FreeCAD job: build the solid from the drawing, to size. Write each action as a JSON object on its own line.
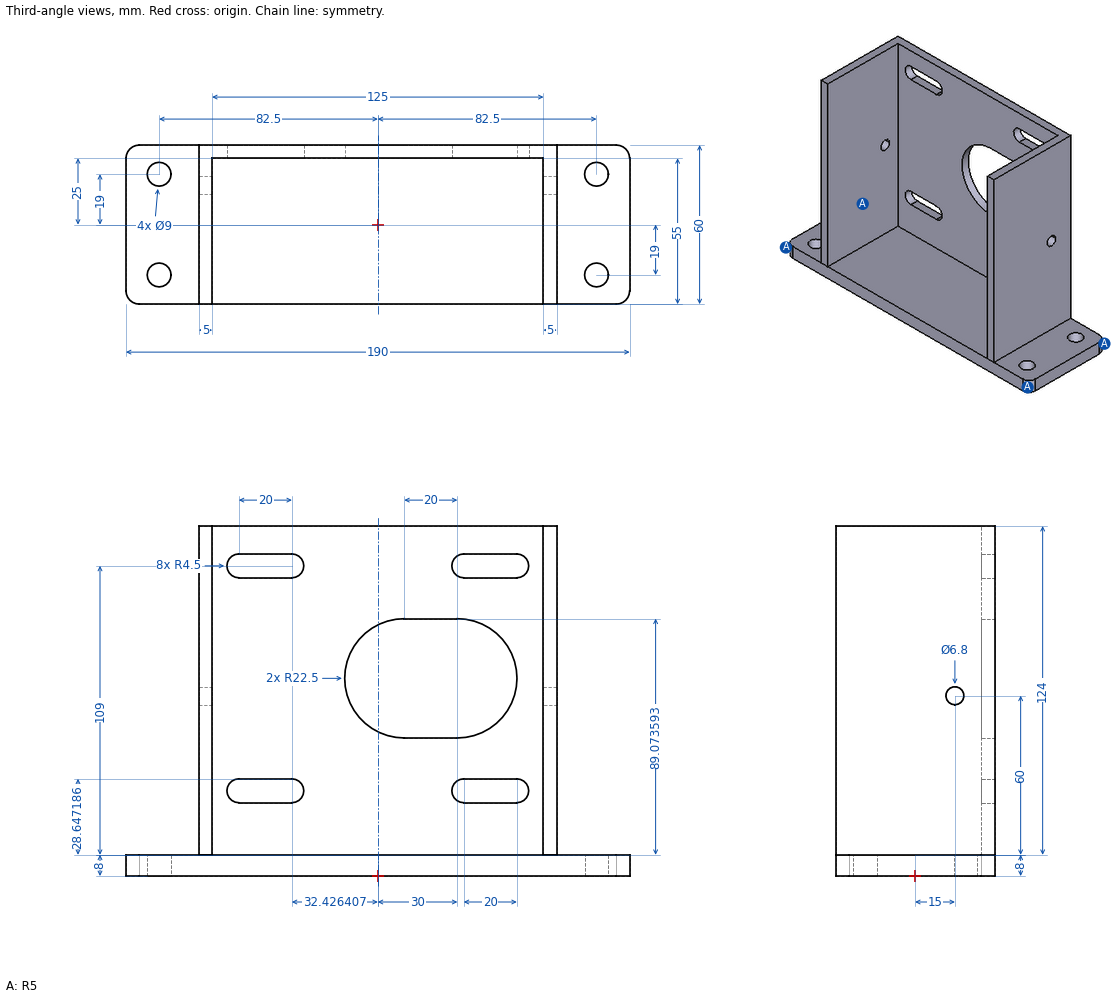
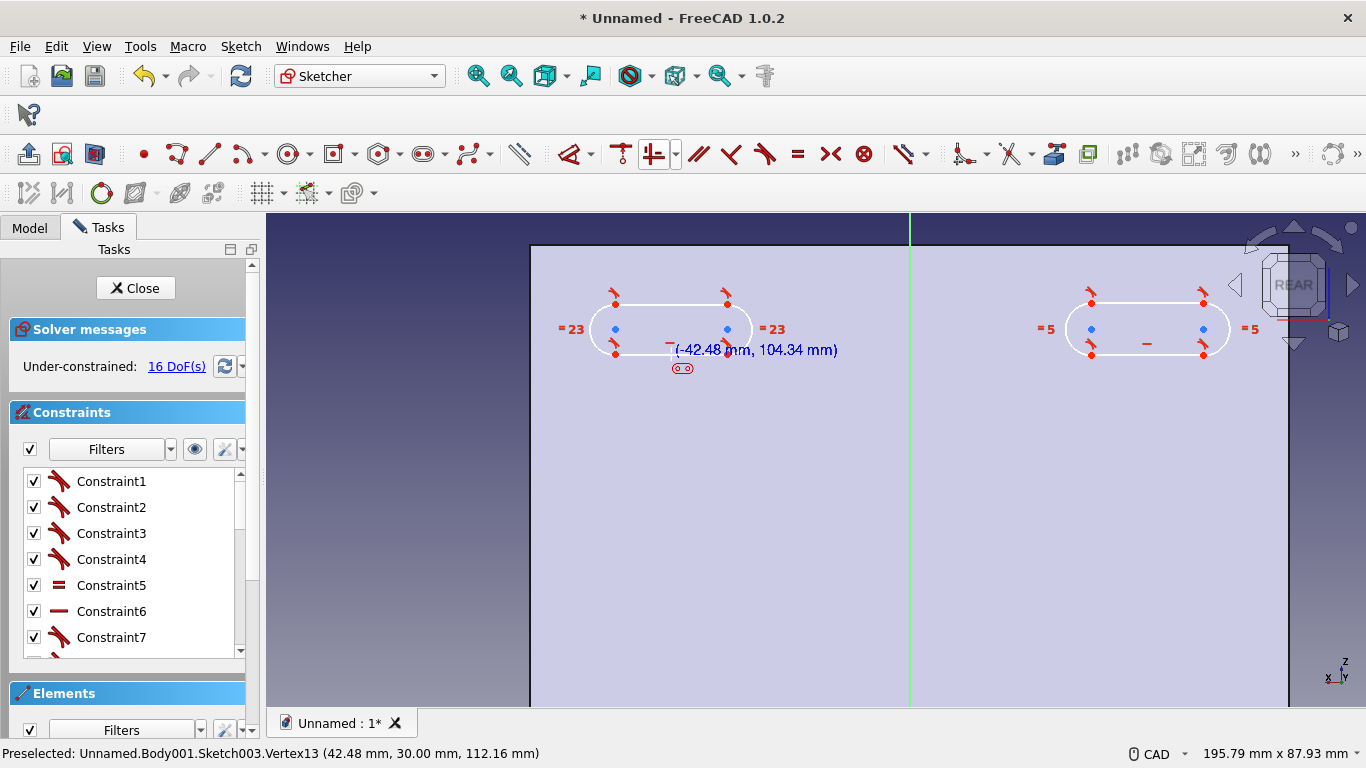
{"action": "left_click", "coordinate": [741, 567]}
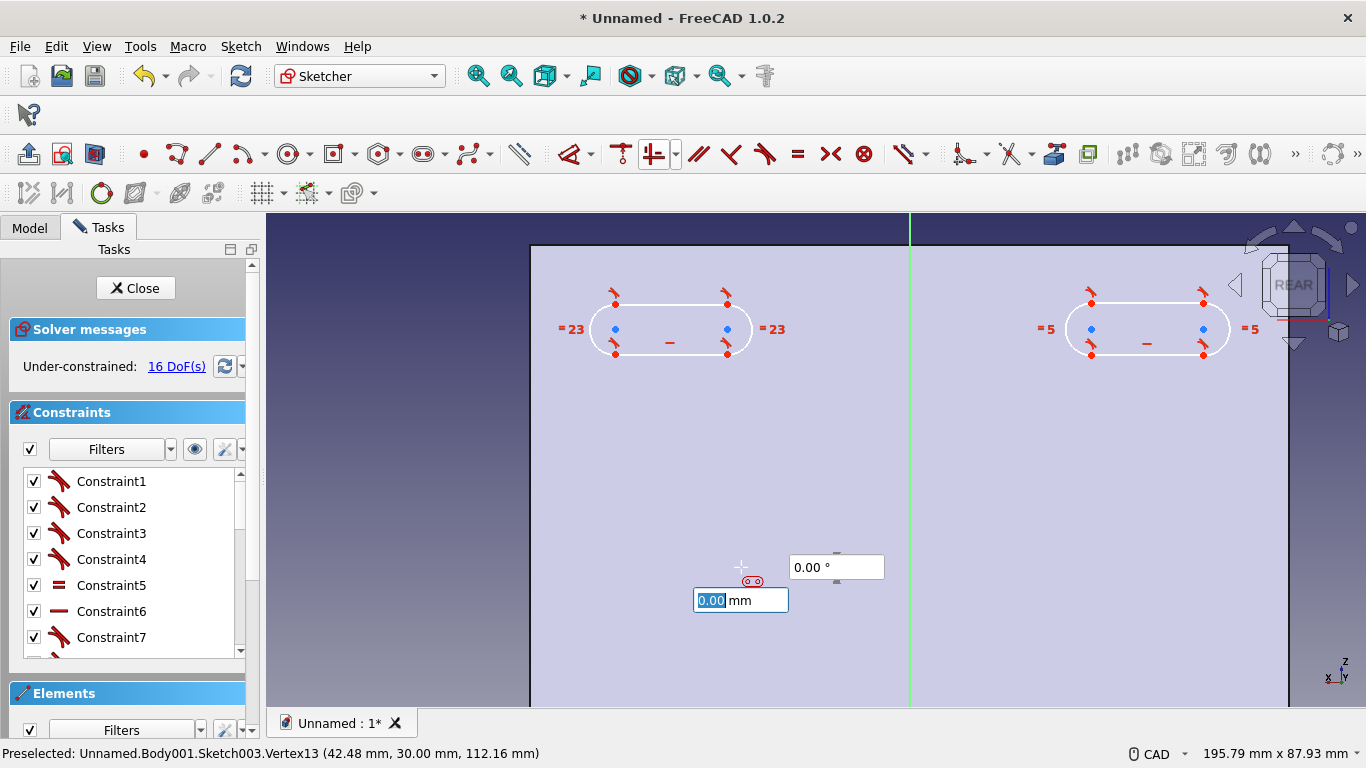
{"action": "left_click", "coordinate": [853, 567]}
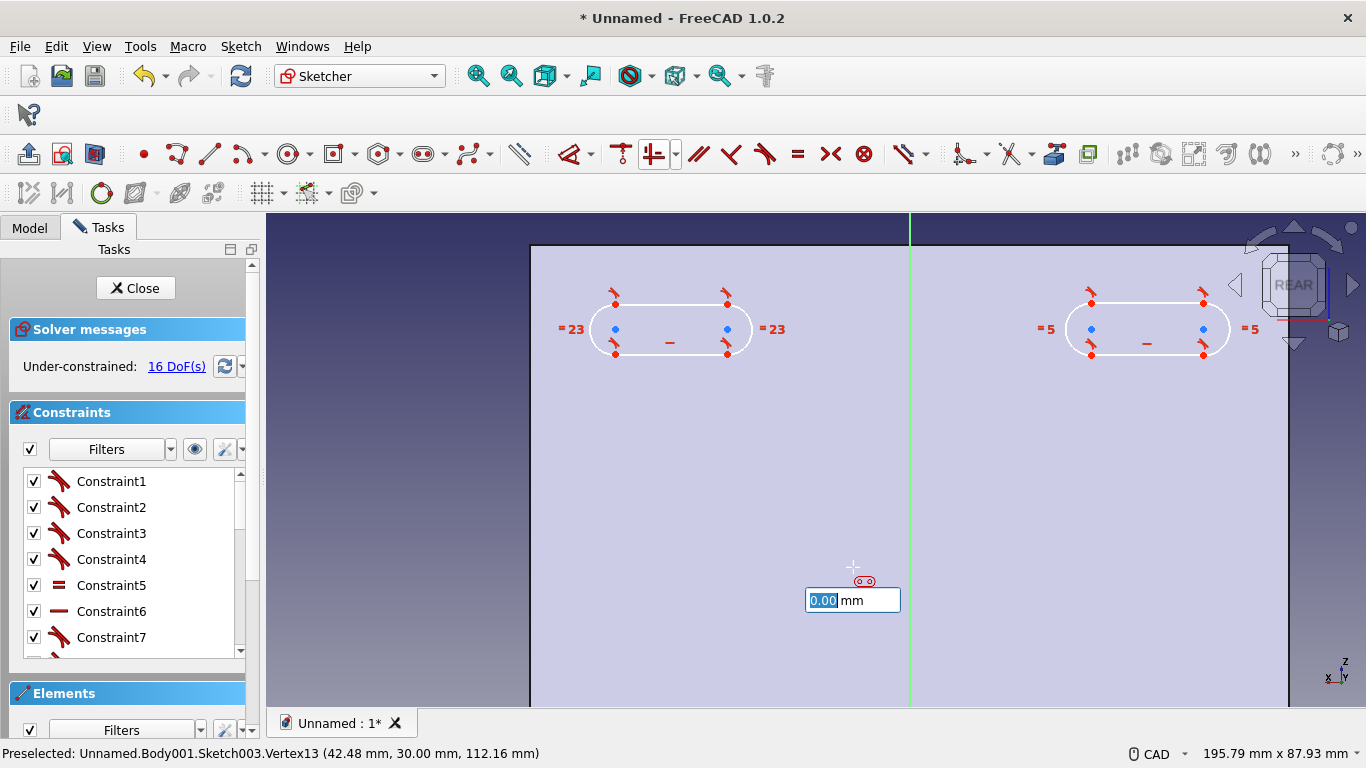
{"action": "scroll", "coordinate": [615, 327], "scroll_direction": "down", "scroll_amount": 4}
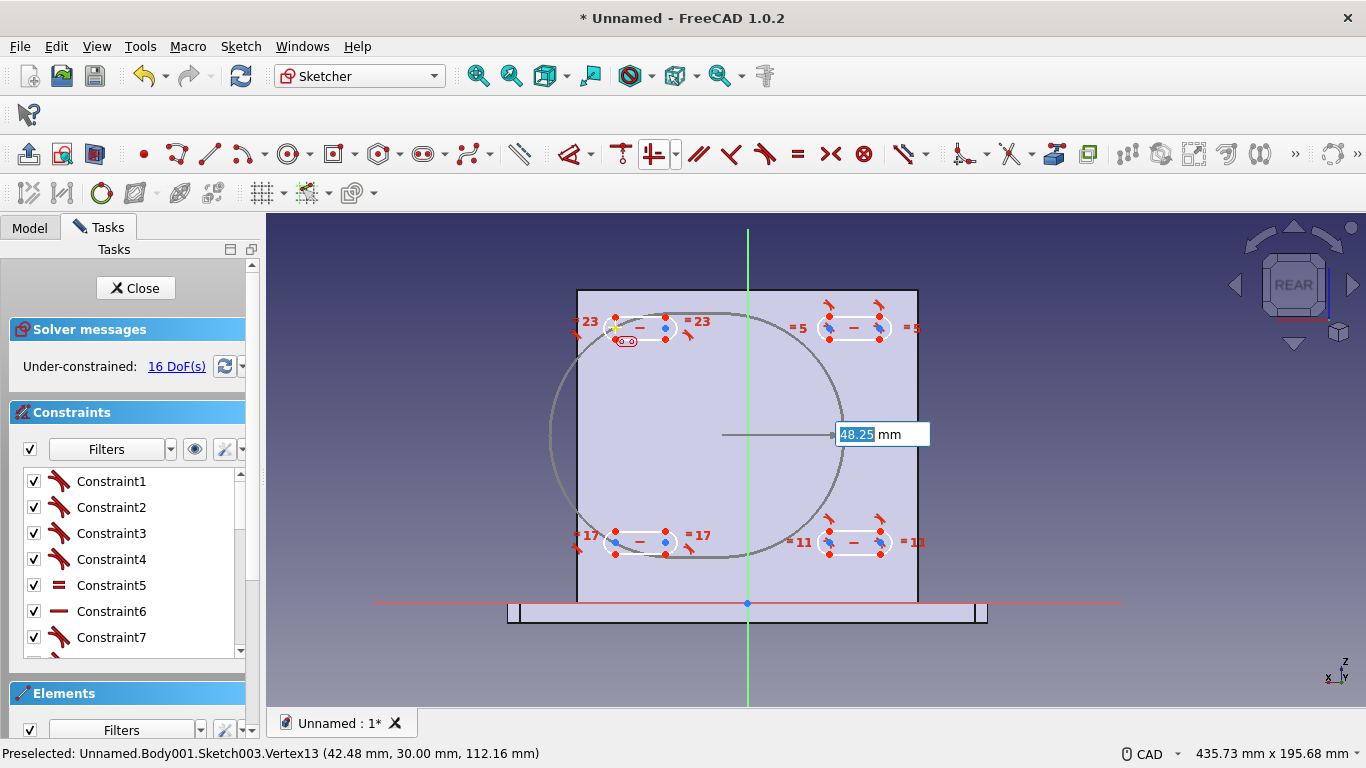
{"action": "left_click", "coordinate": [697, 492]}
{"action": "key", "text": "Escape"}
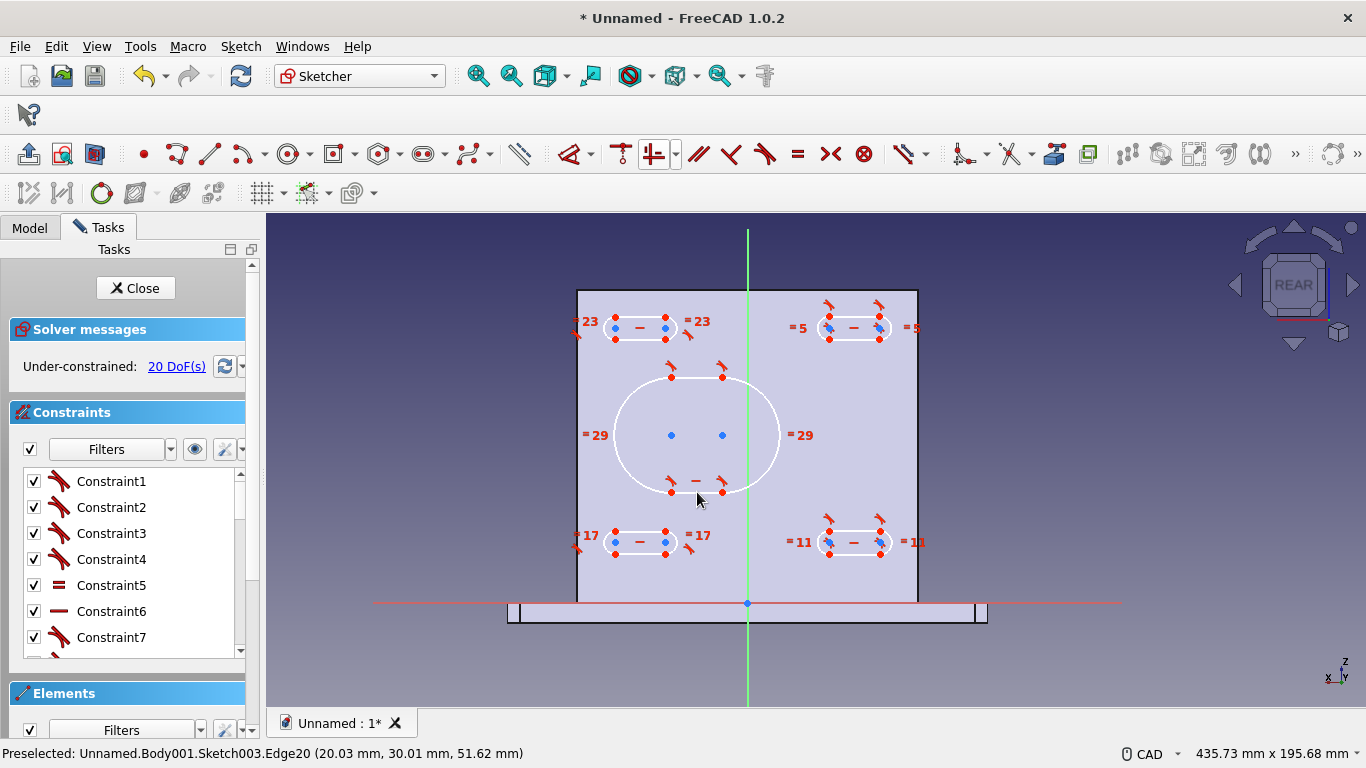
{"action": "scroll", "coordinate": [820, 321], "scroll_direction": "up", "scroll_amount": 2}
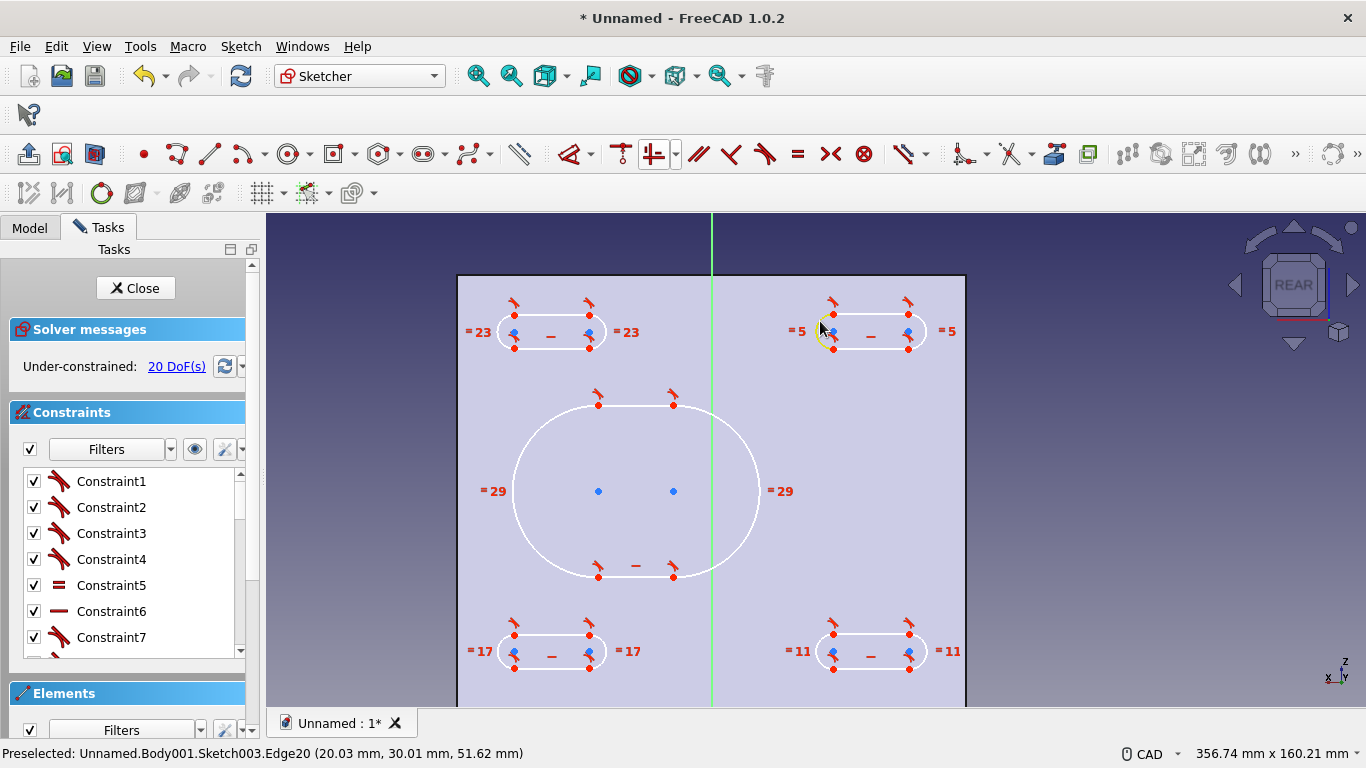
{"action": "left_click", "coordinate": [820, 321]}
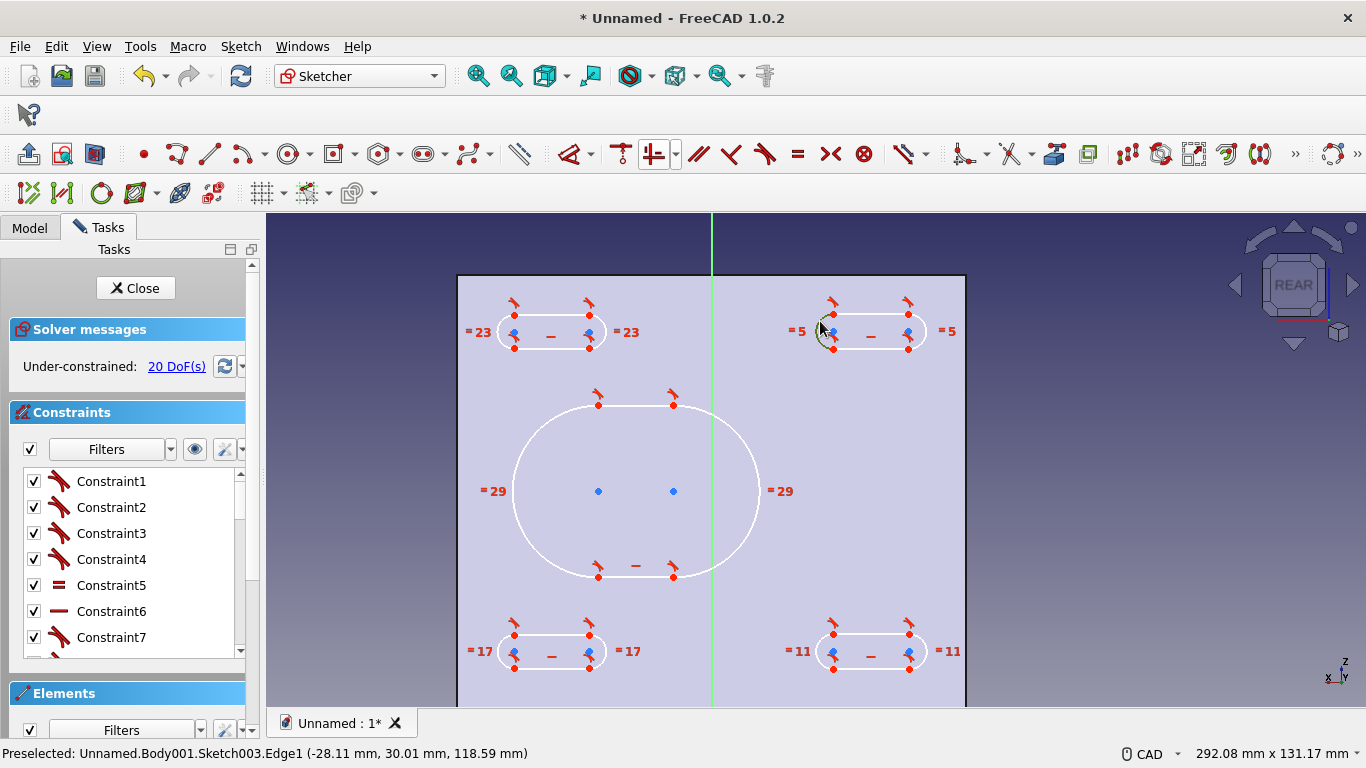
{"action": "left_click", "coordinate": [819, 642]}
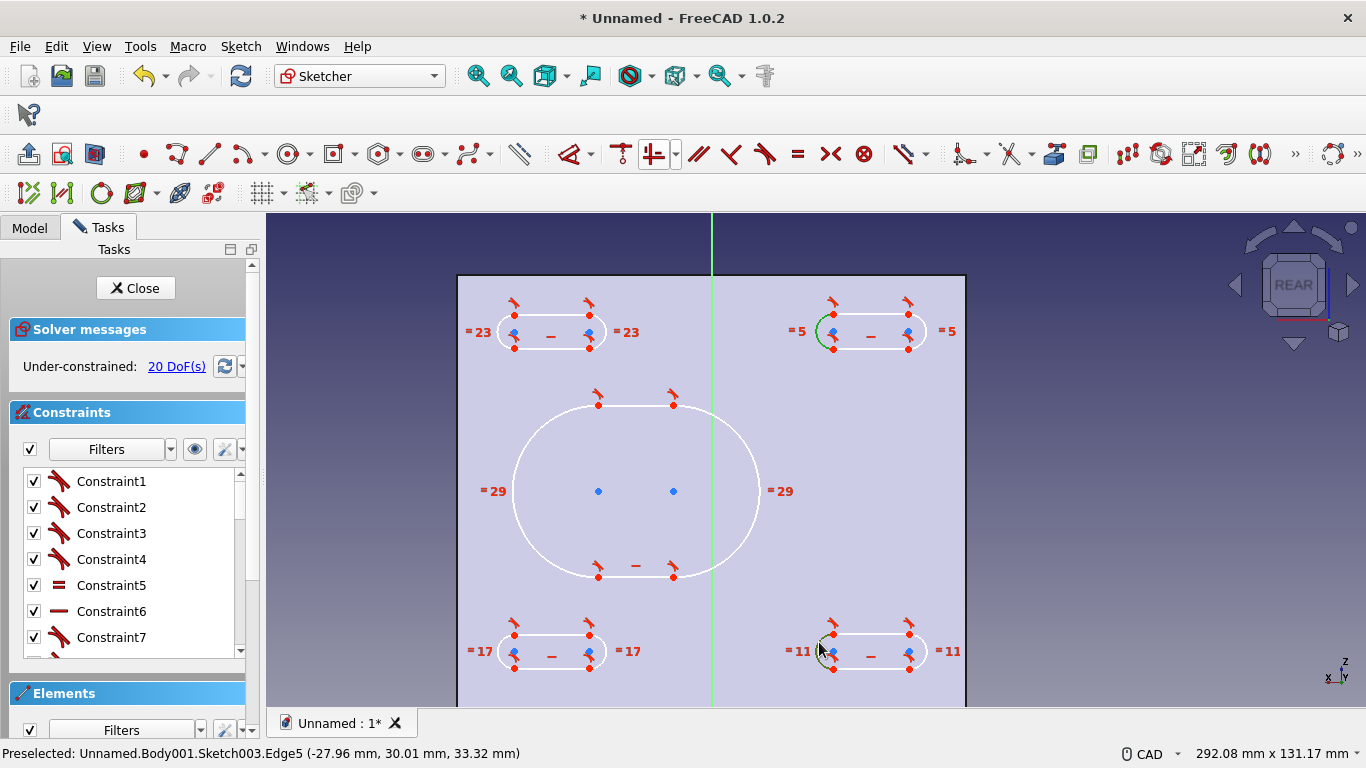
{"action": "left_click", "coordinate": [501, 642]}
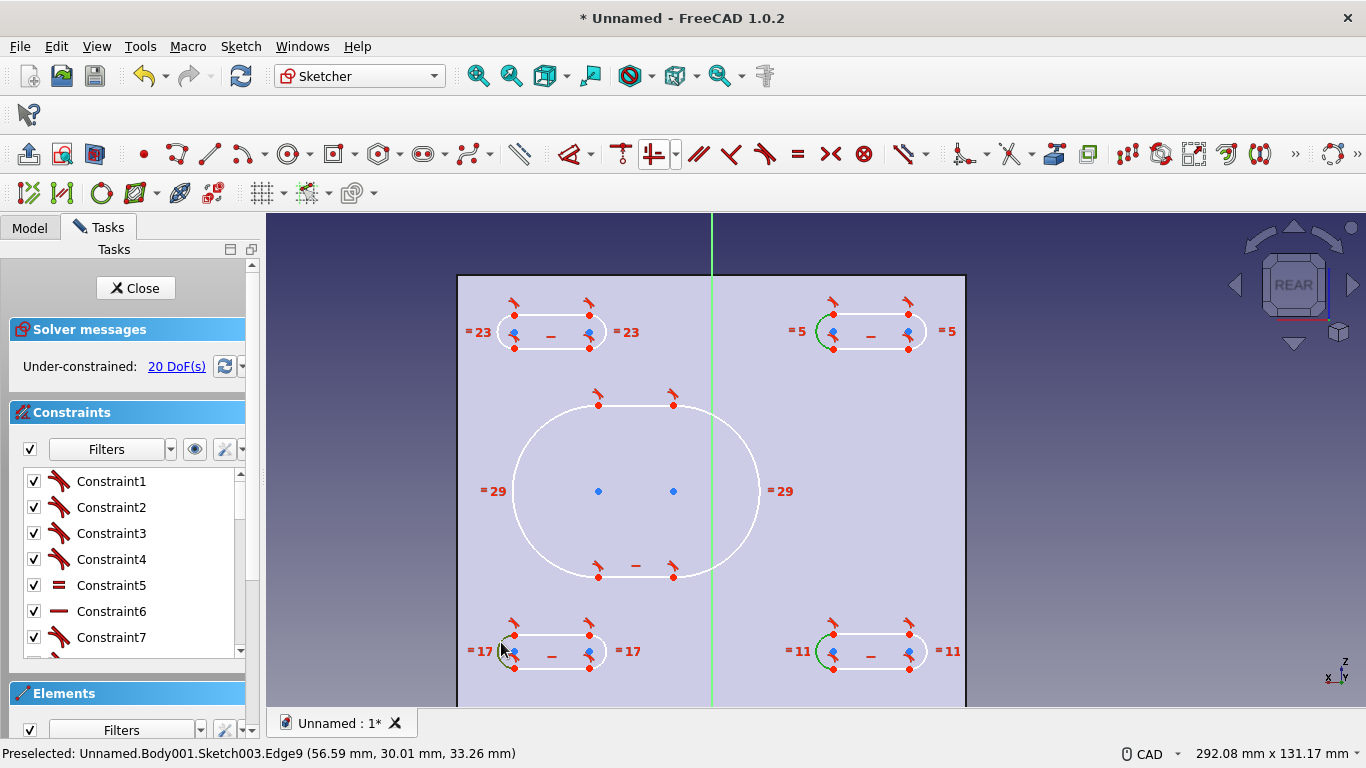
{"action": "left_click", "coordinate": [501, 322]}